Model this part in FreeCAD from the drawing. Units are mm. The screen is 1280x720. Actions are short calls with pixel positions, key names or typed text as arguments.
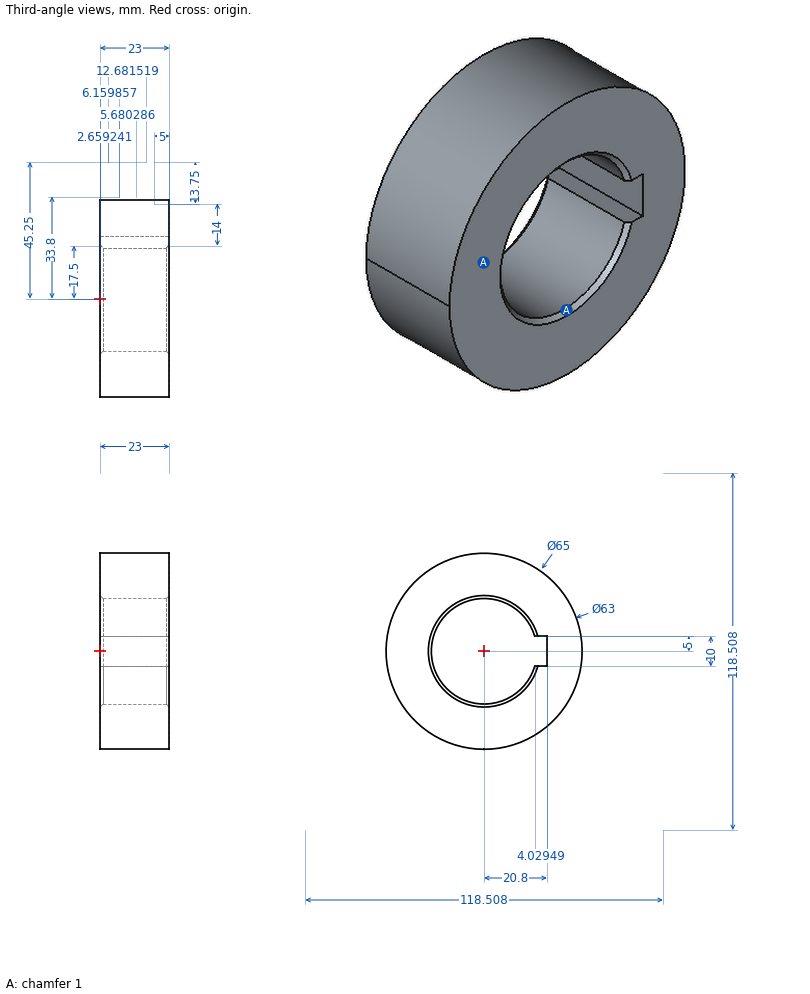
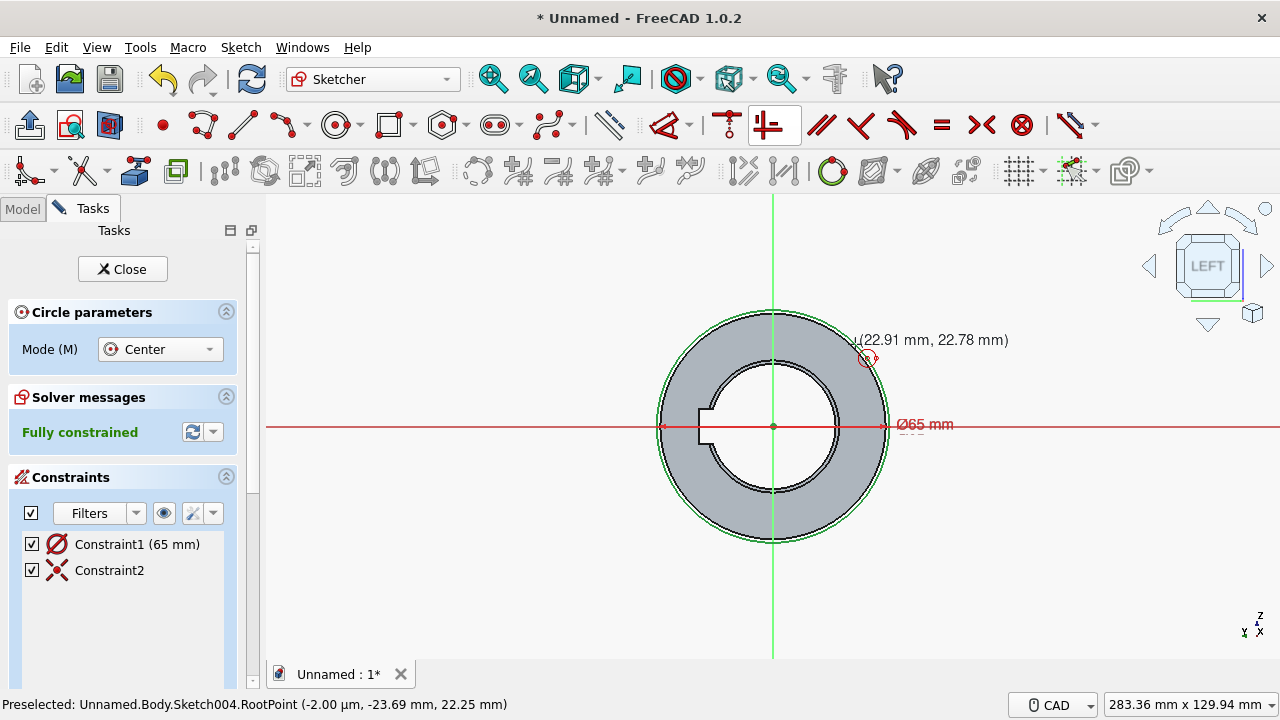
click(773, 427)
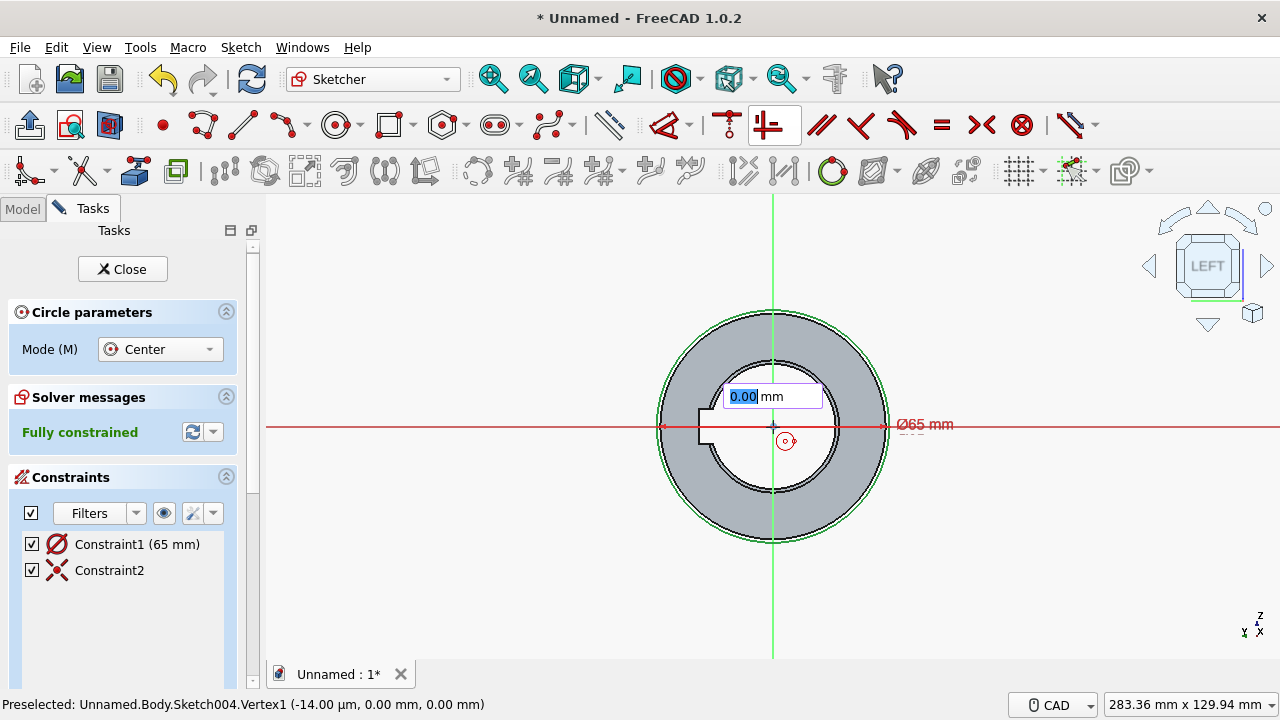
scroll(853, 347, up, 8)
move(849, 345)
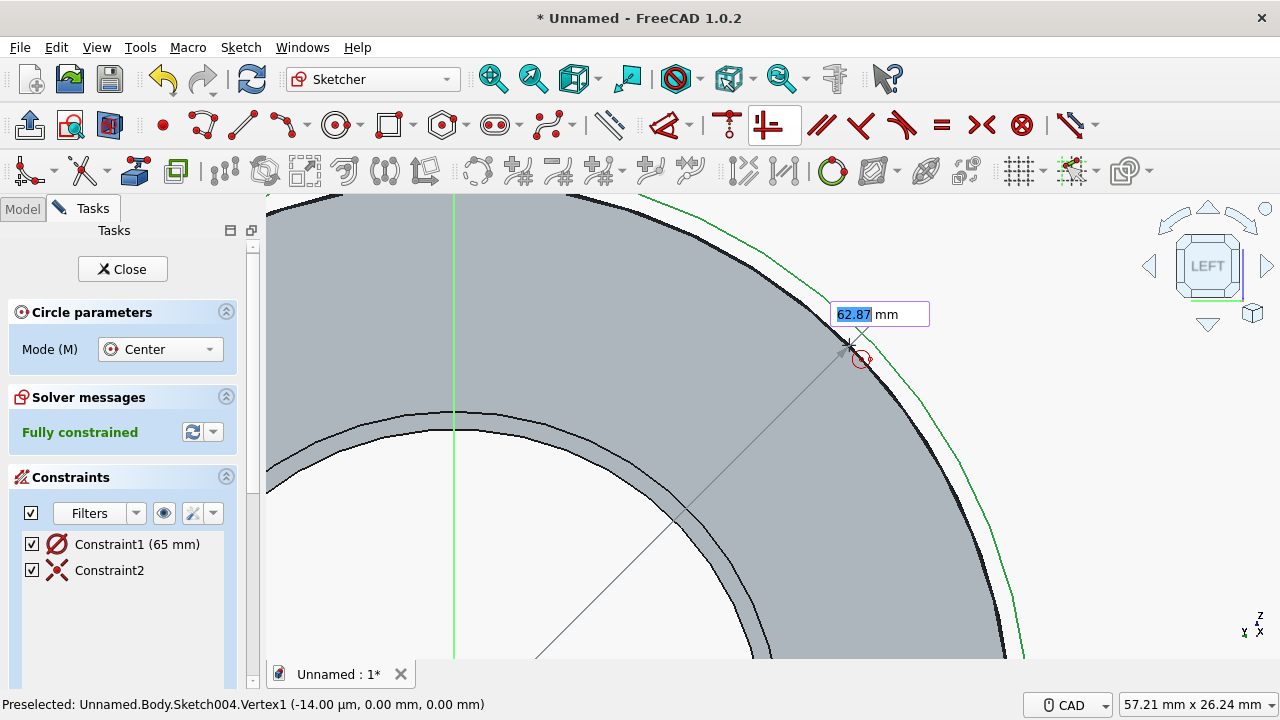
text(63)
key(Return)
key(Escape)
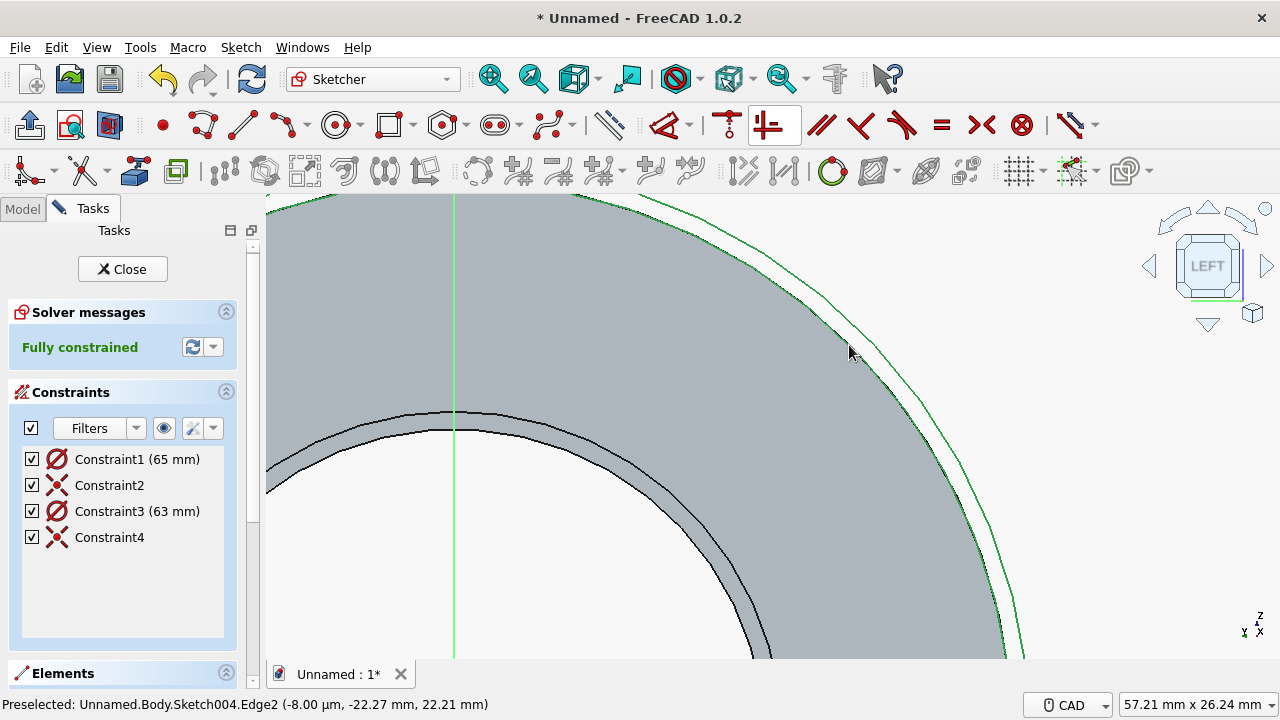
click(123, 269)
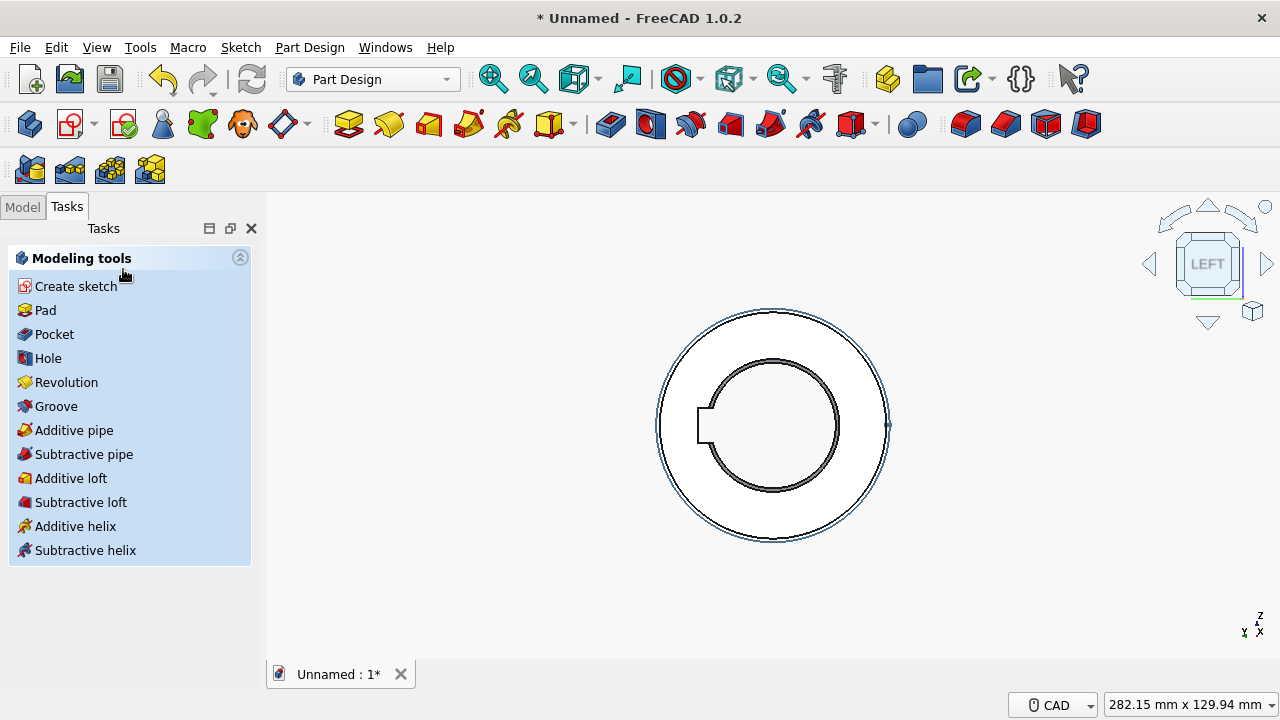
click(350, 124)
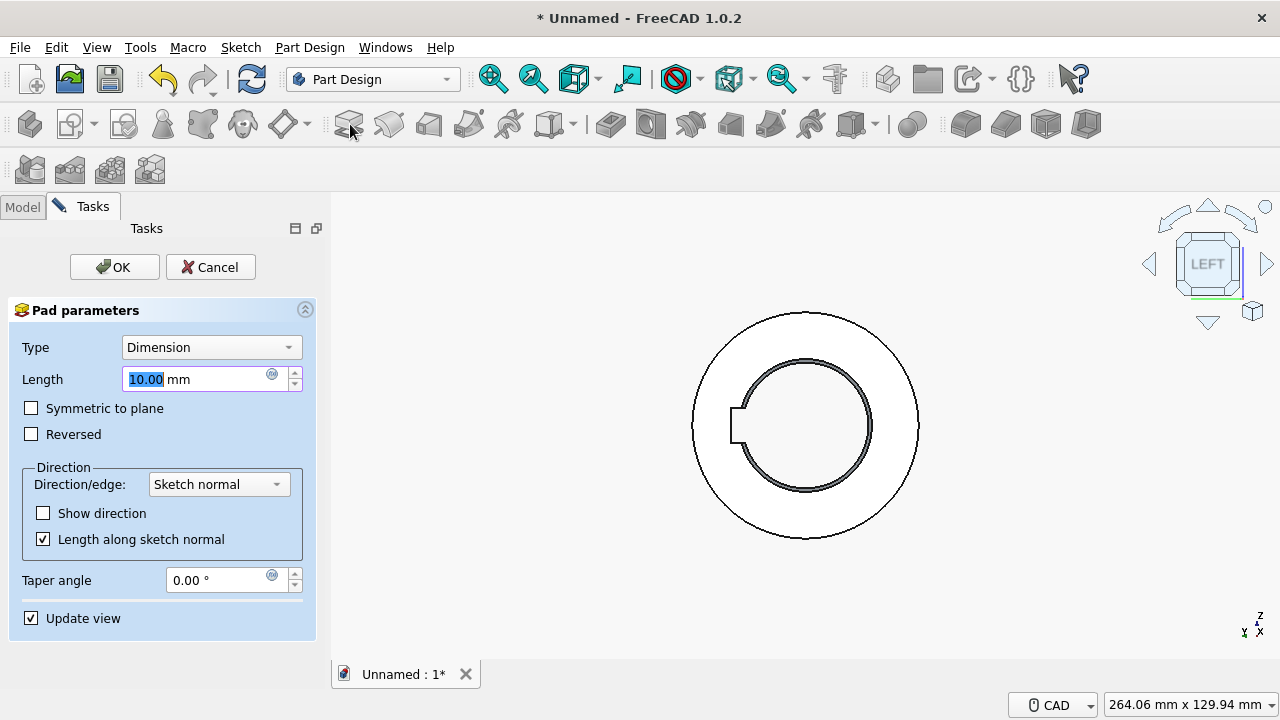
text(23)
key(Tab)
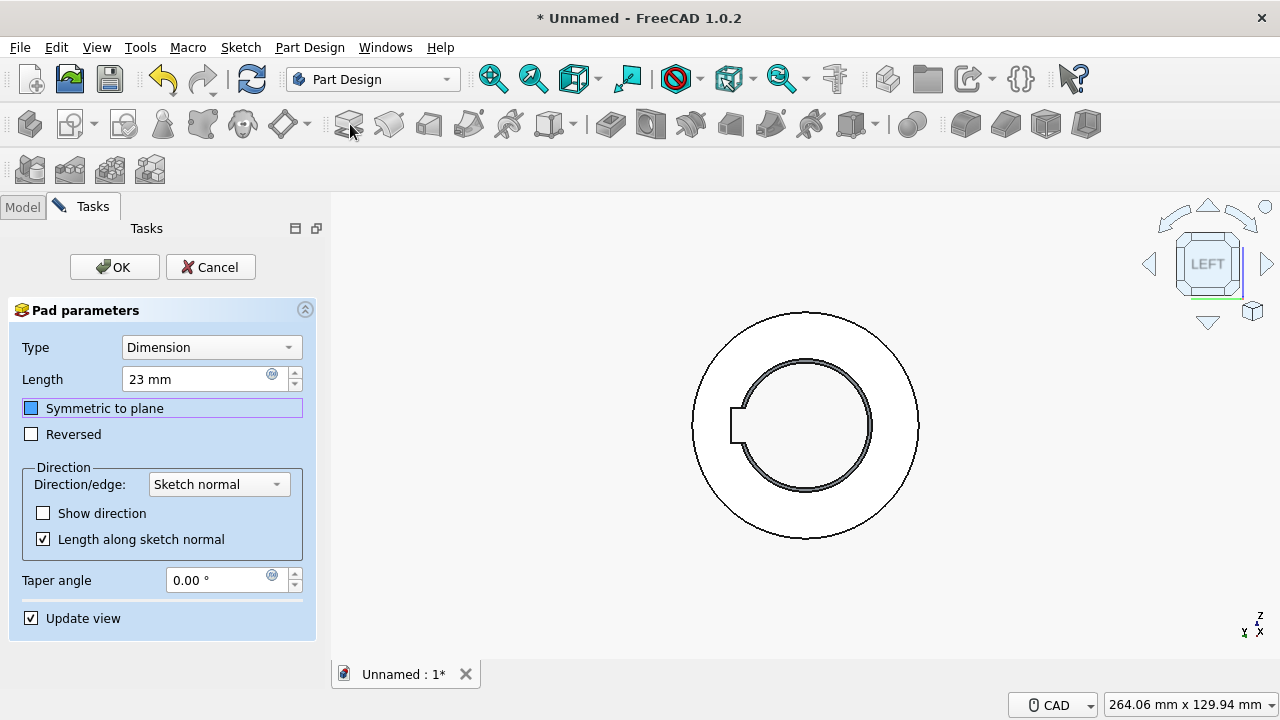
click(30, 434)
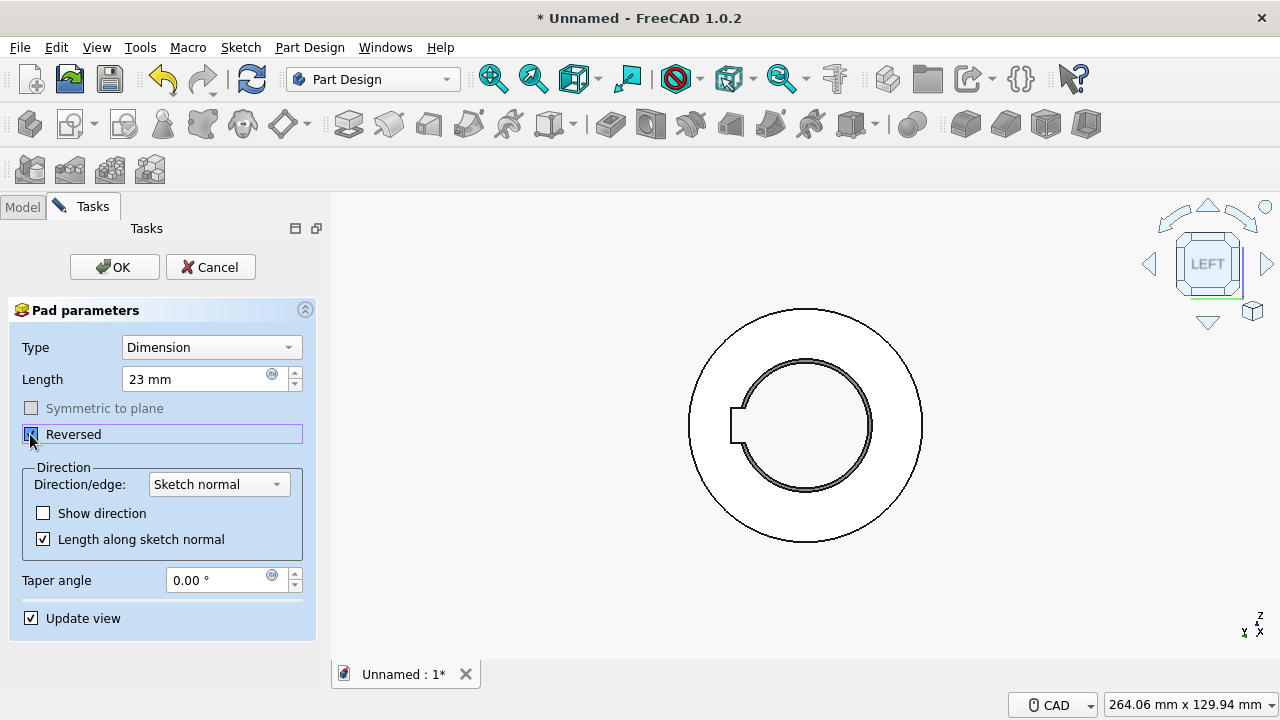
click(115, 267)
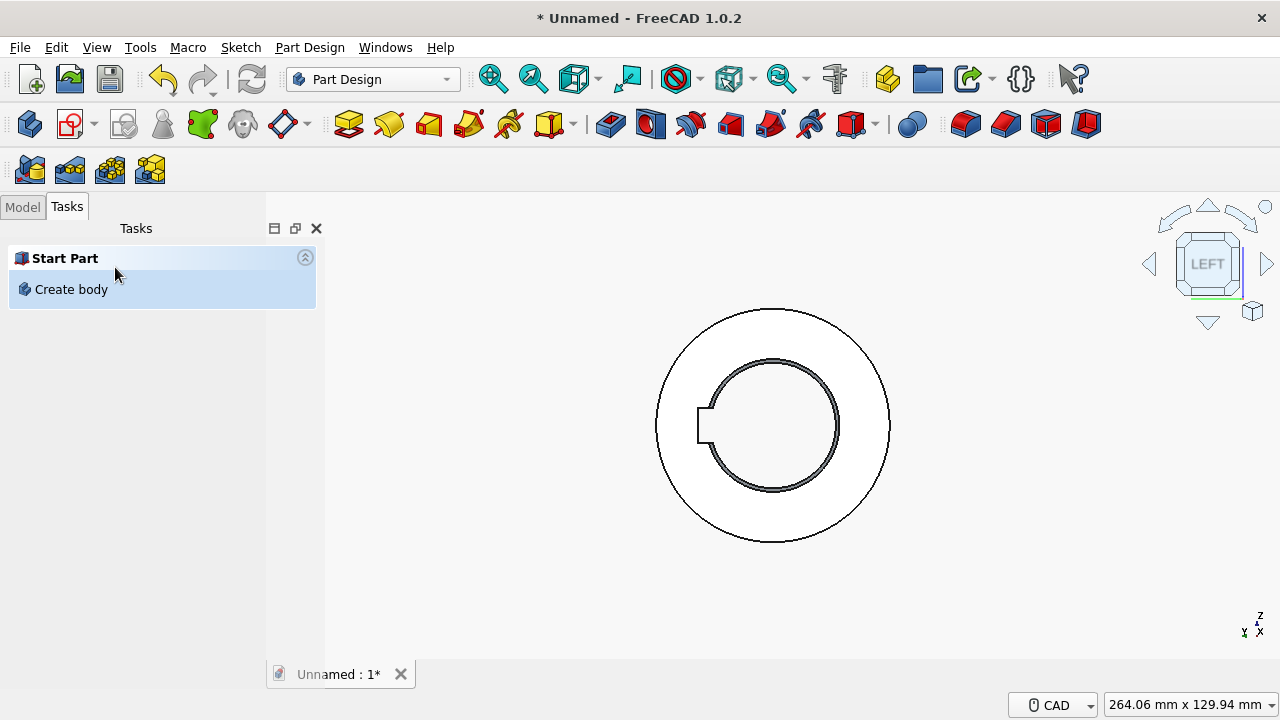
key(0)